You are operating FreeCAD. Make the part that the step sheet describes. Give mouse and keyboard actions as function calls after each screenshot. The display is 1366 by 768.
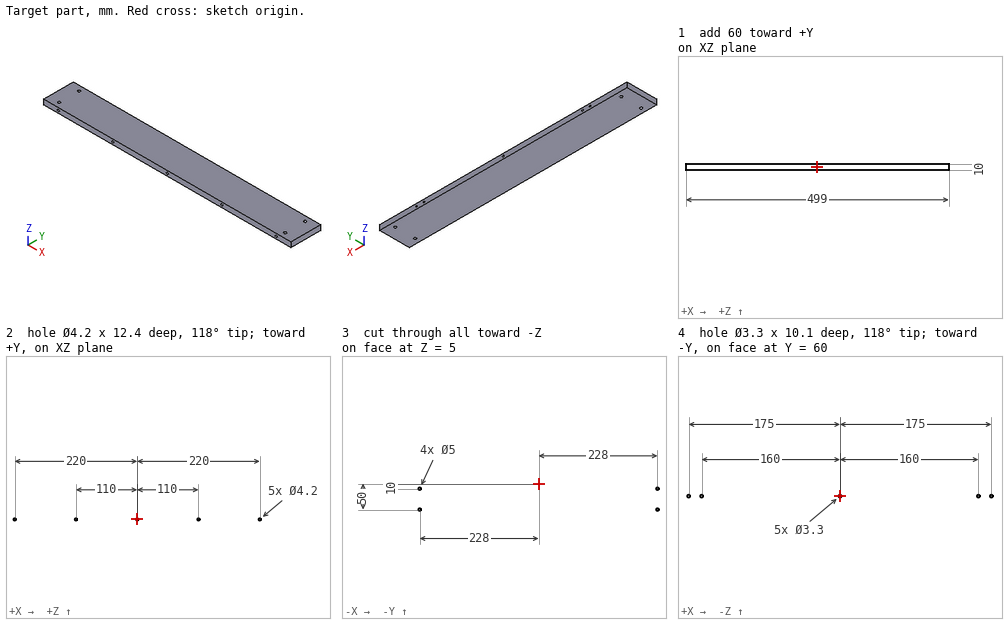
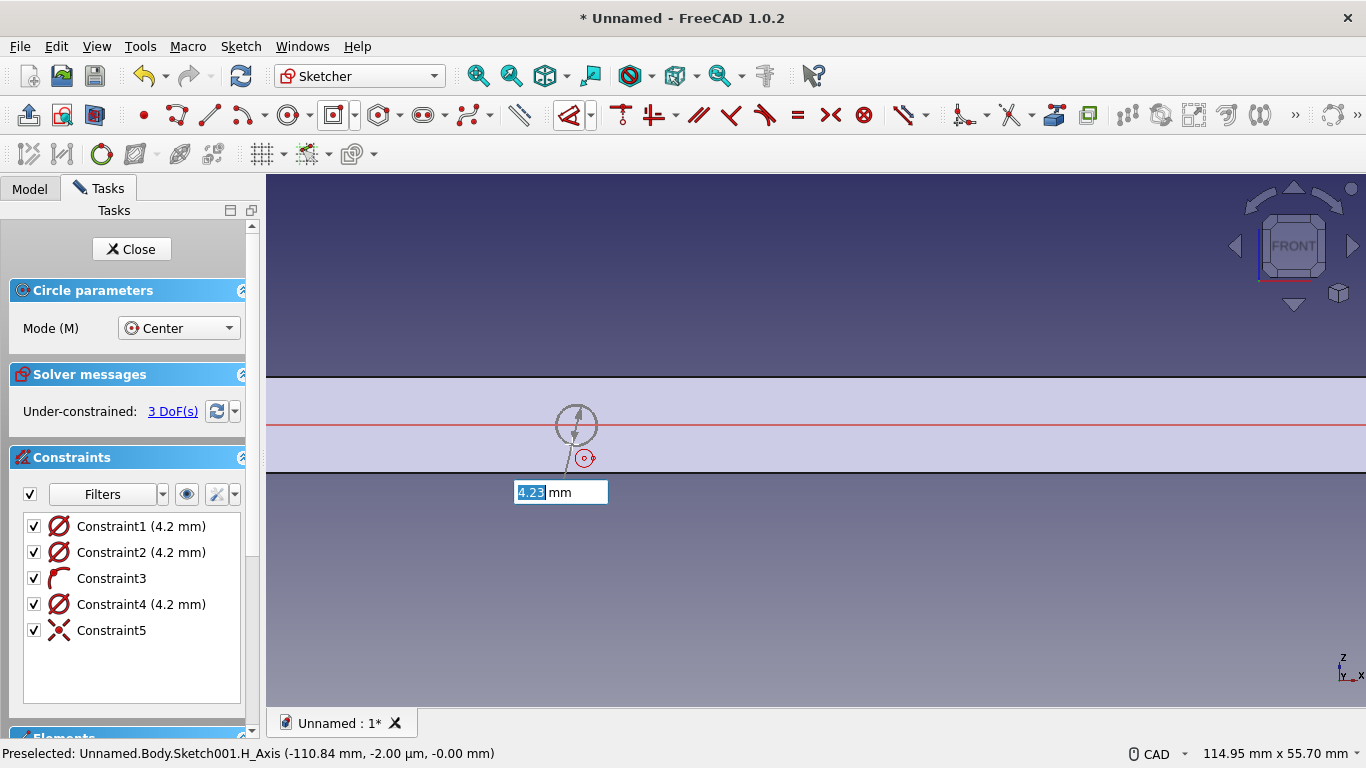
text(4.2)
key(Return)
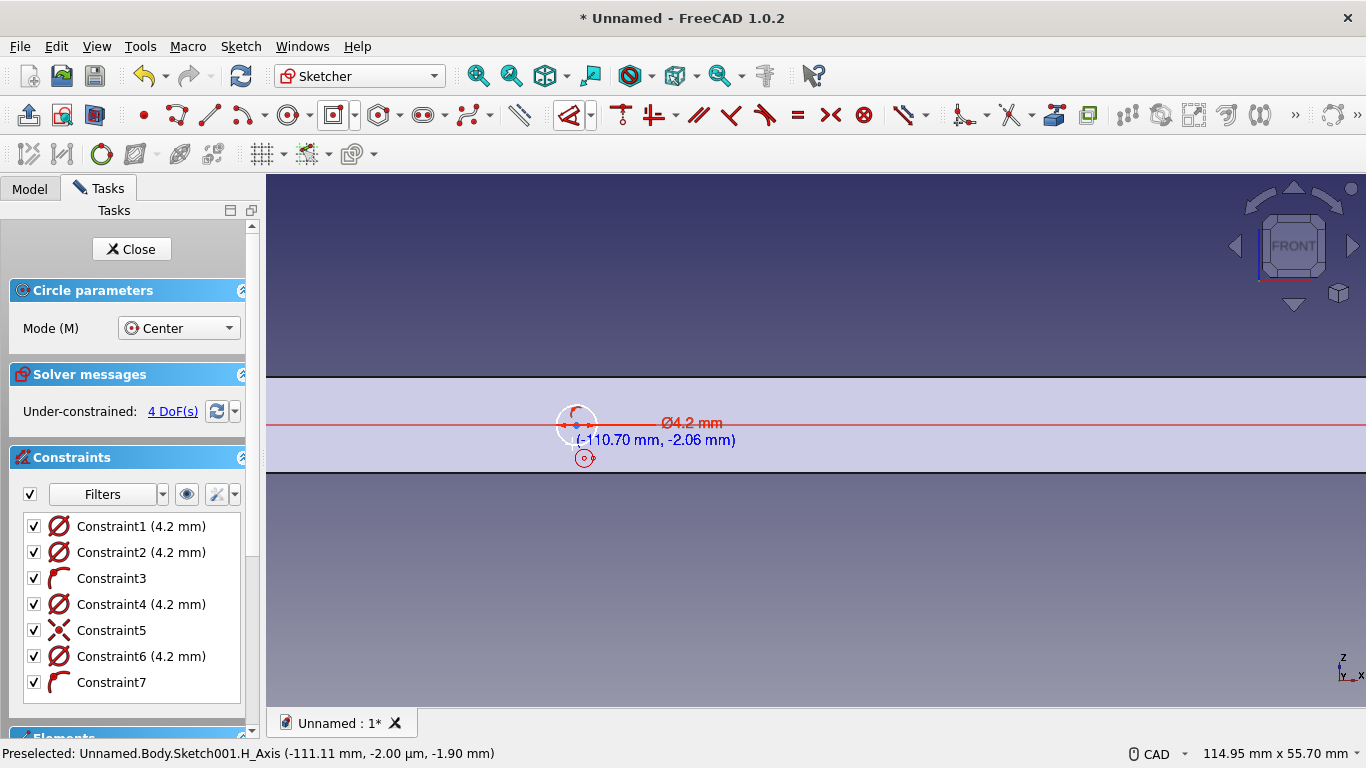
scroll(572, 444, down, 9)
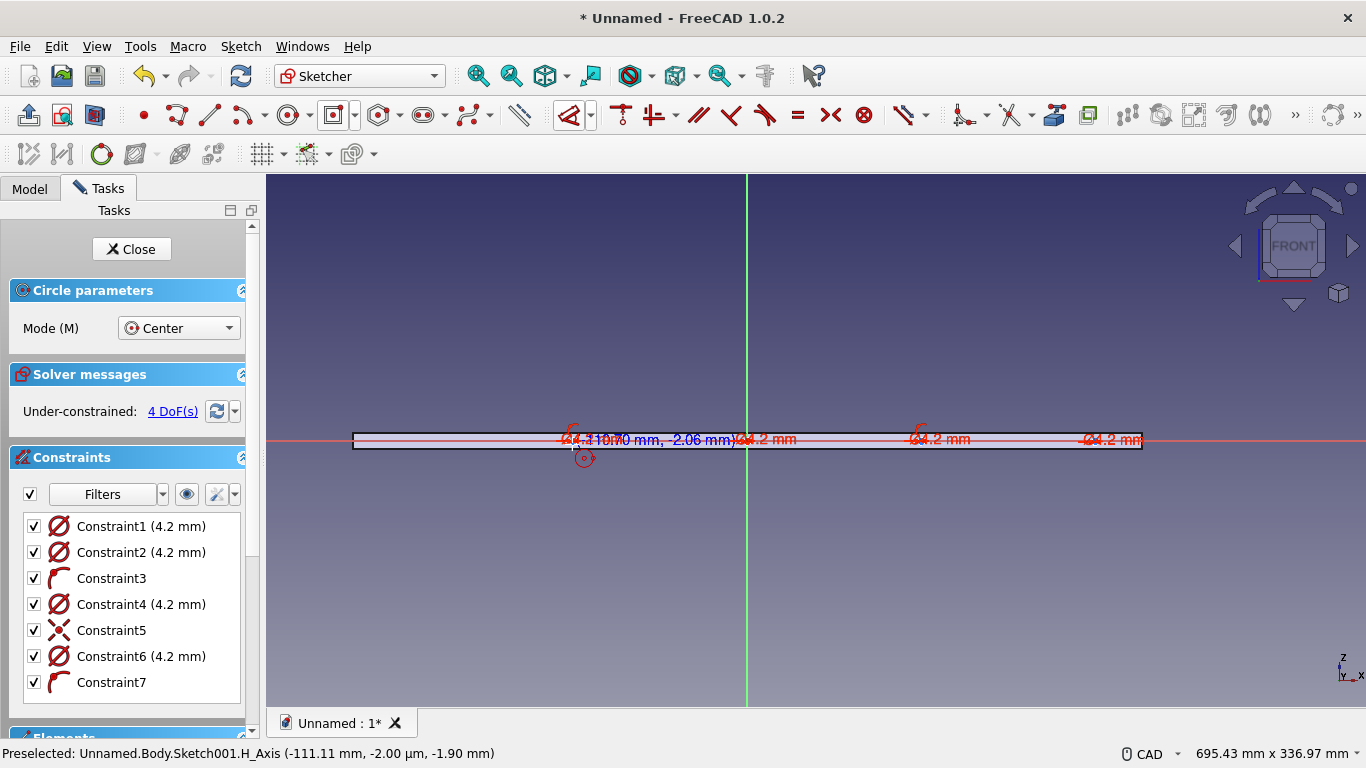
scroll(399, 441, up, 10)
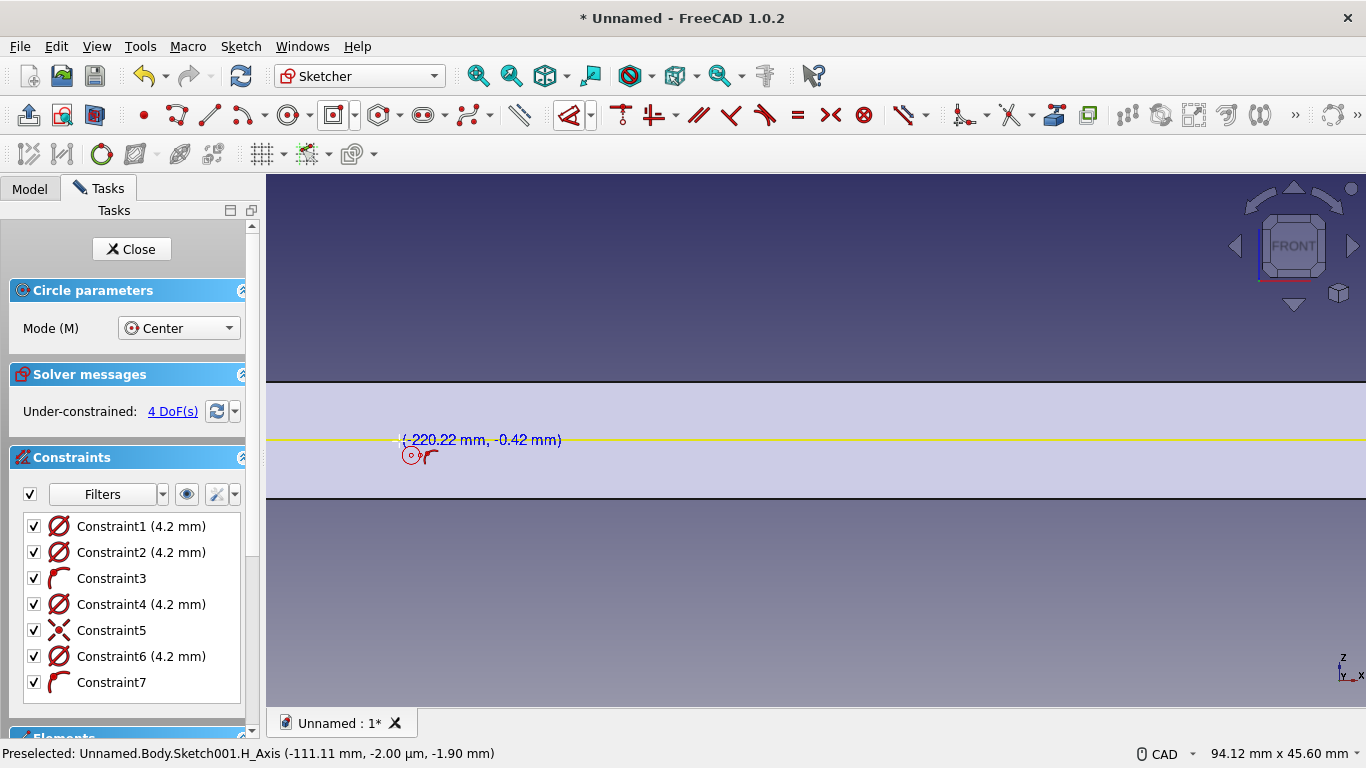
scroll(399, 441, down, 10)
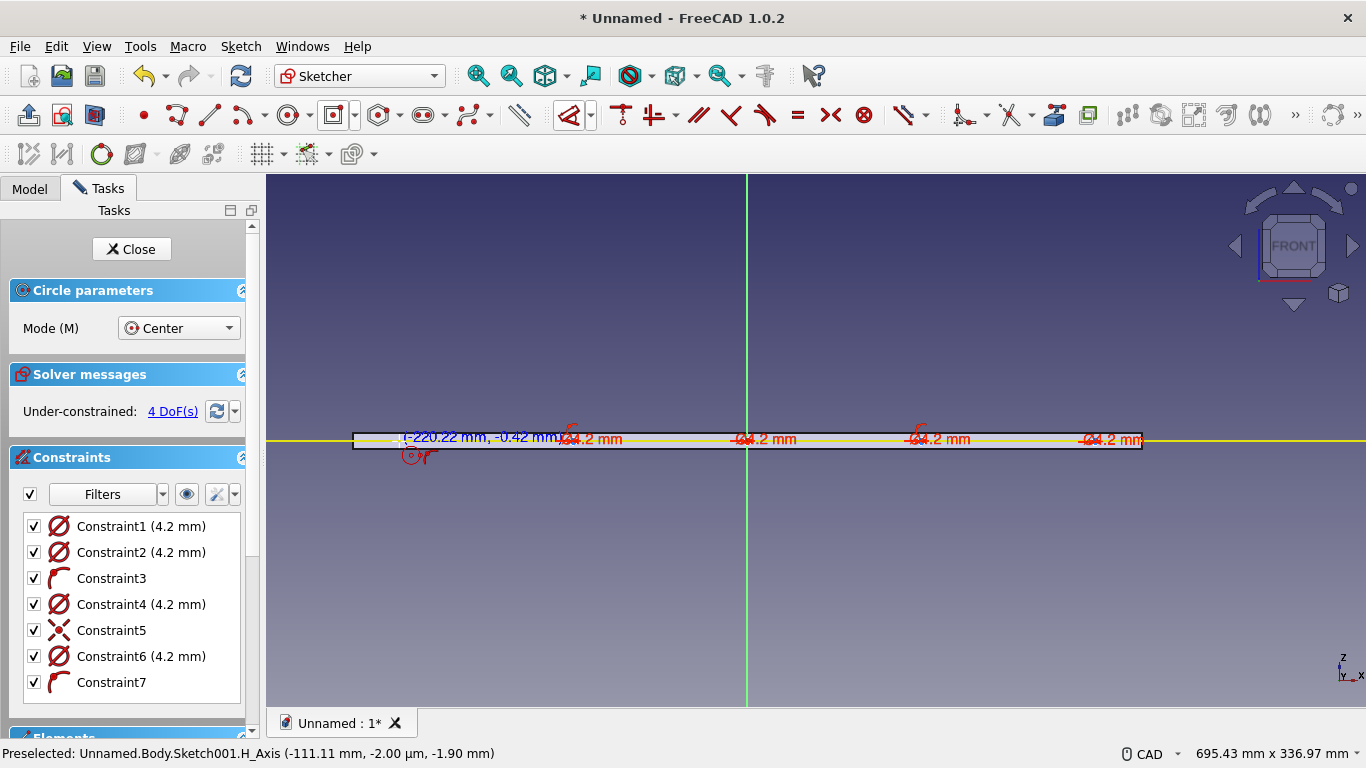
click(399, 441)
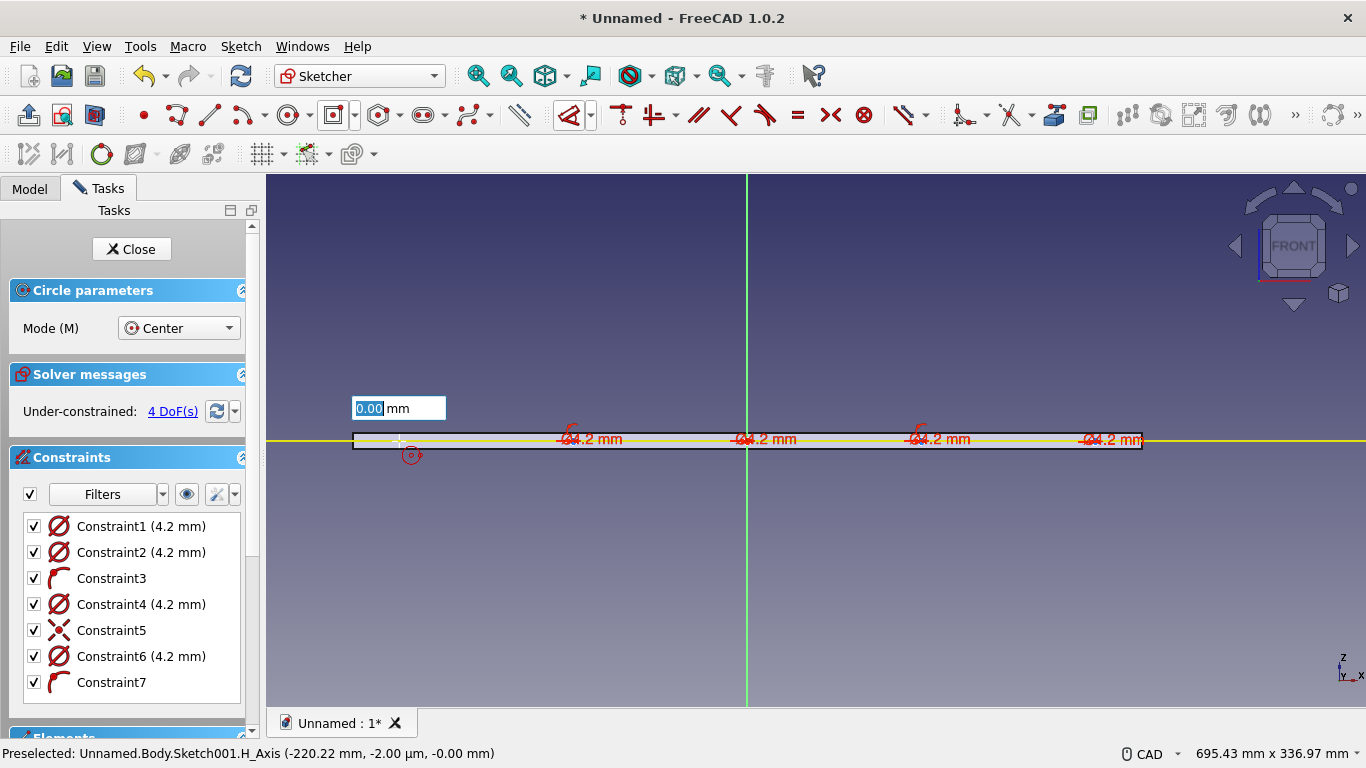
scroll(398, 444, up, 9)
move(399, 444)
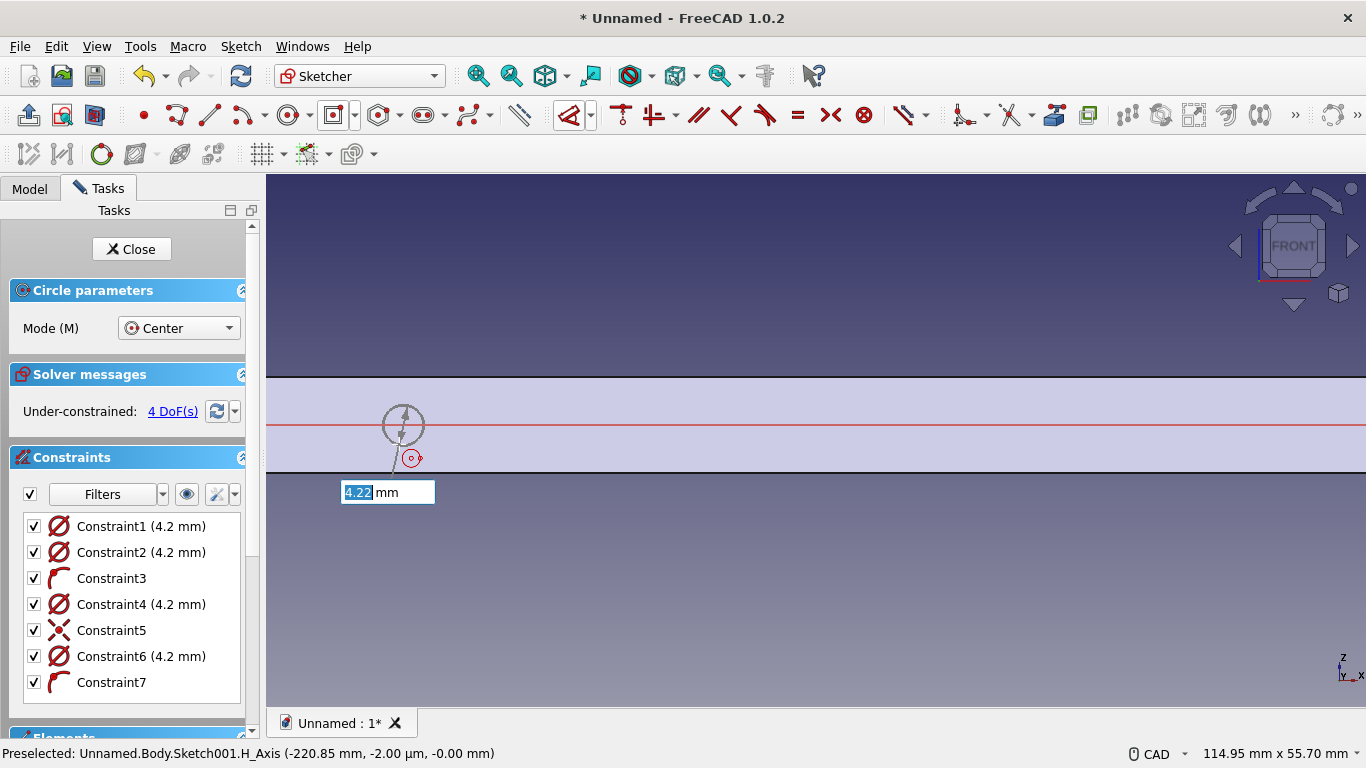
text(4.2)
key(Return)
key(Escape)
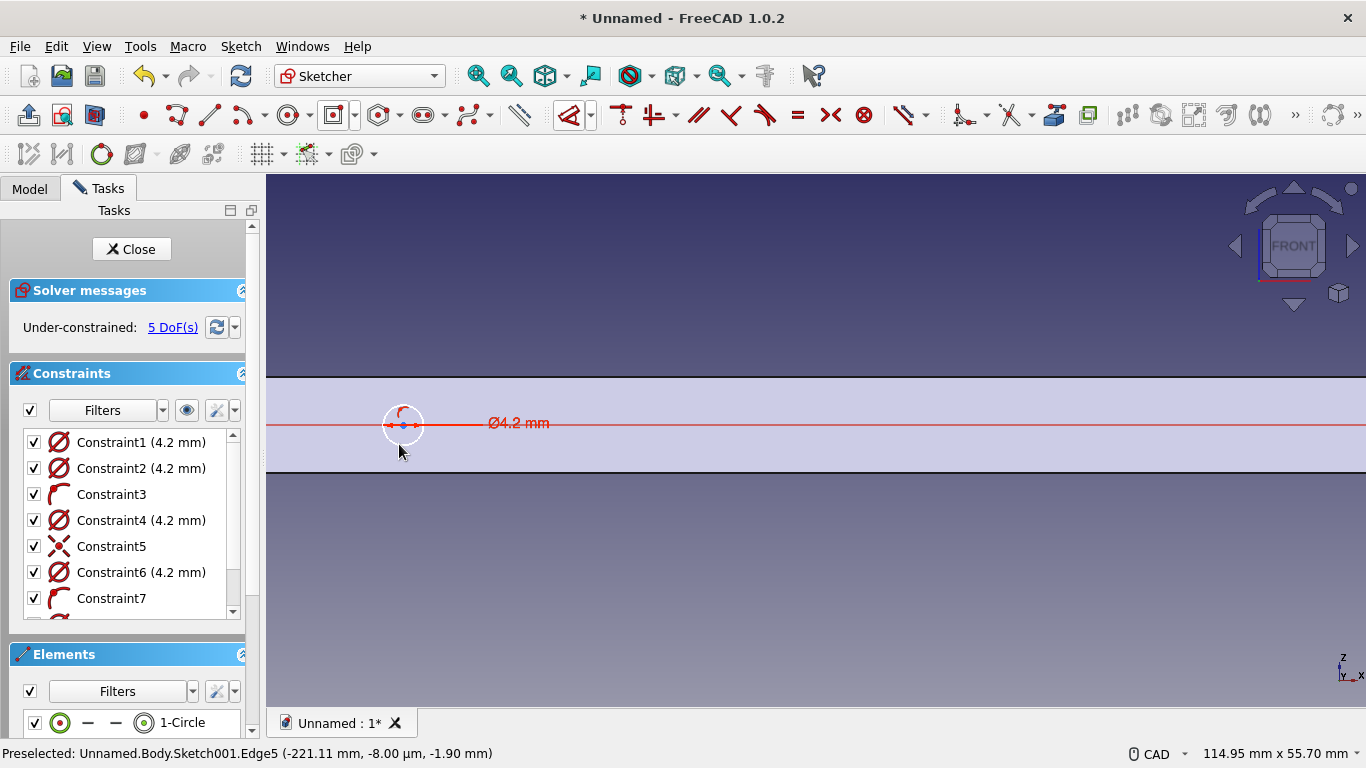
scroll(398, 444, down, 9)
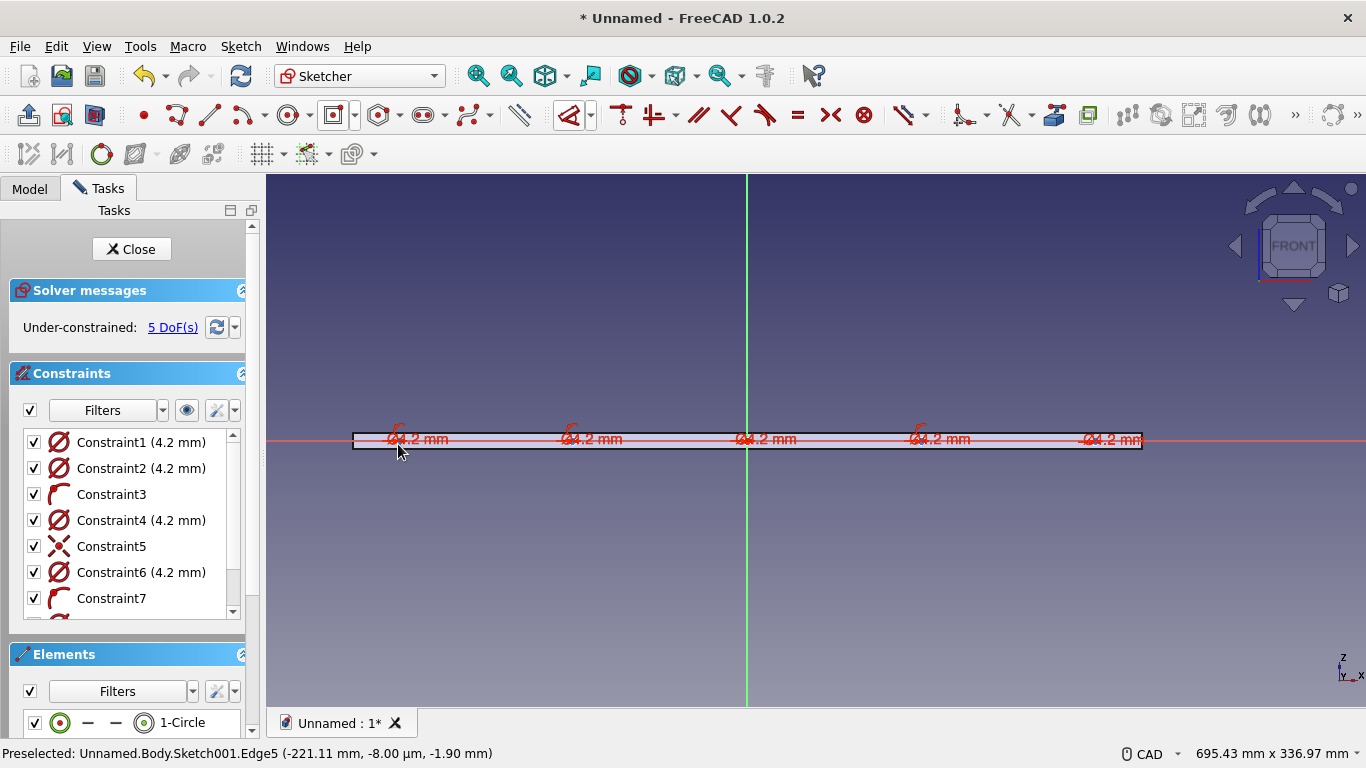
click(1095, 442)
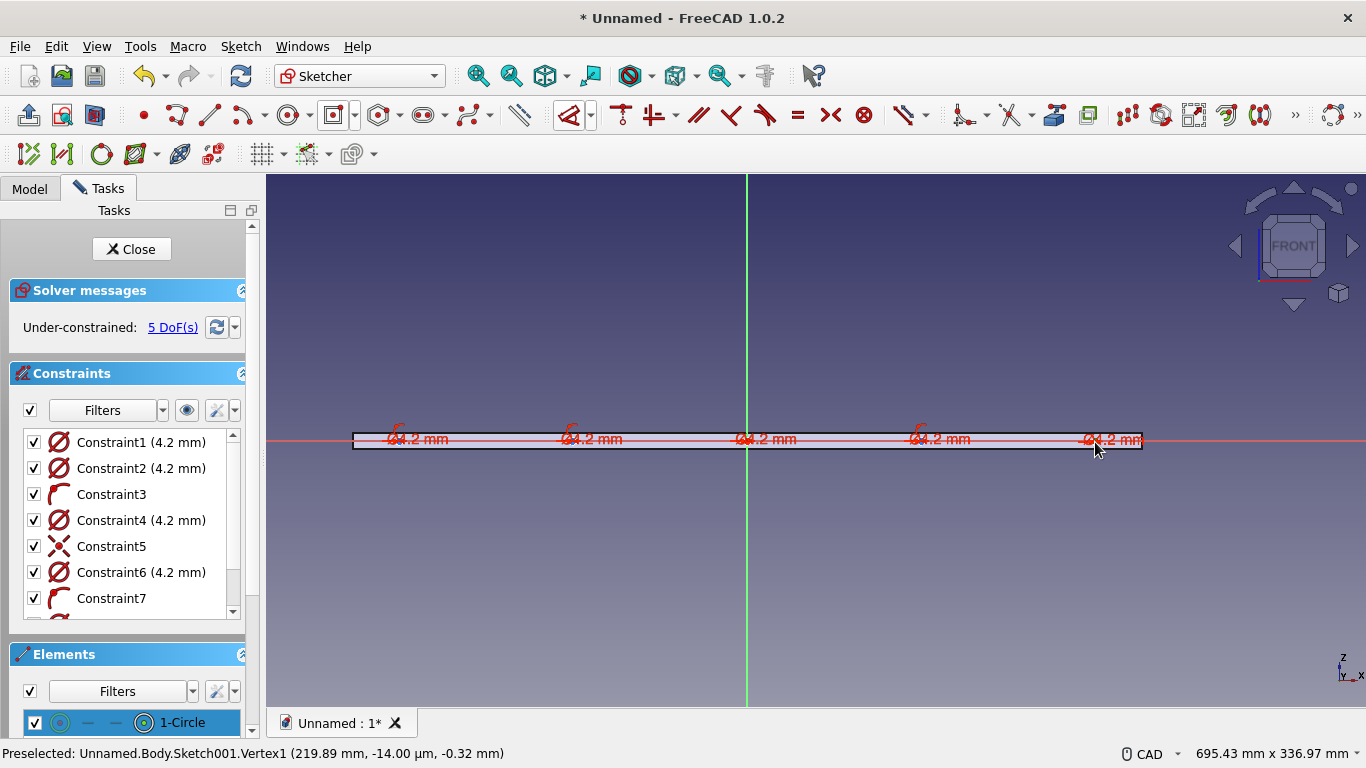
click(359, 441)